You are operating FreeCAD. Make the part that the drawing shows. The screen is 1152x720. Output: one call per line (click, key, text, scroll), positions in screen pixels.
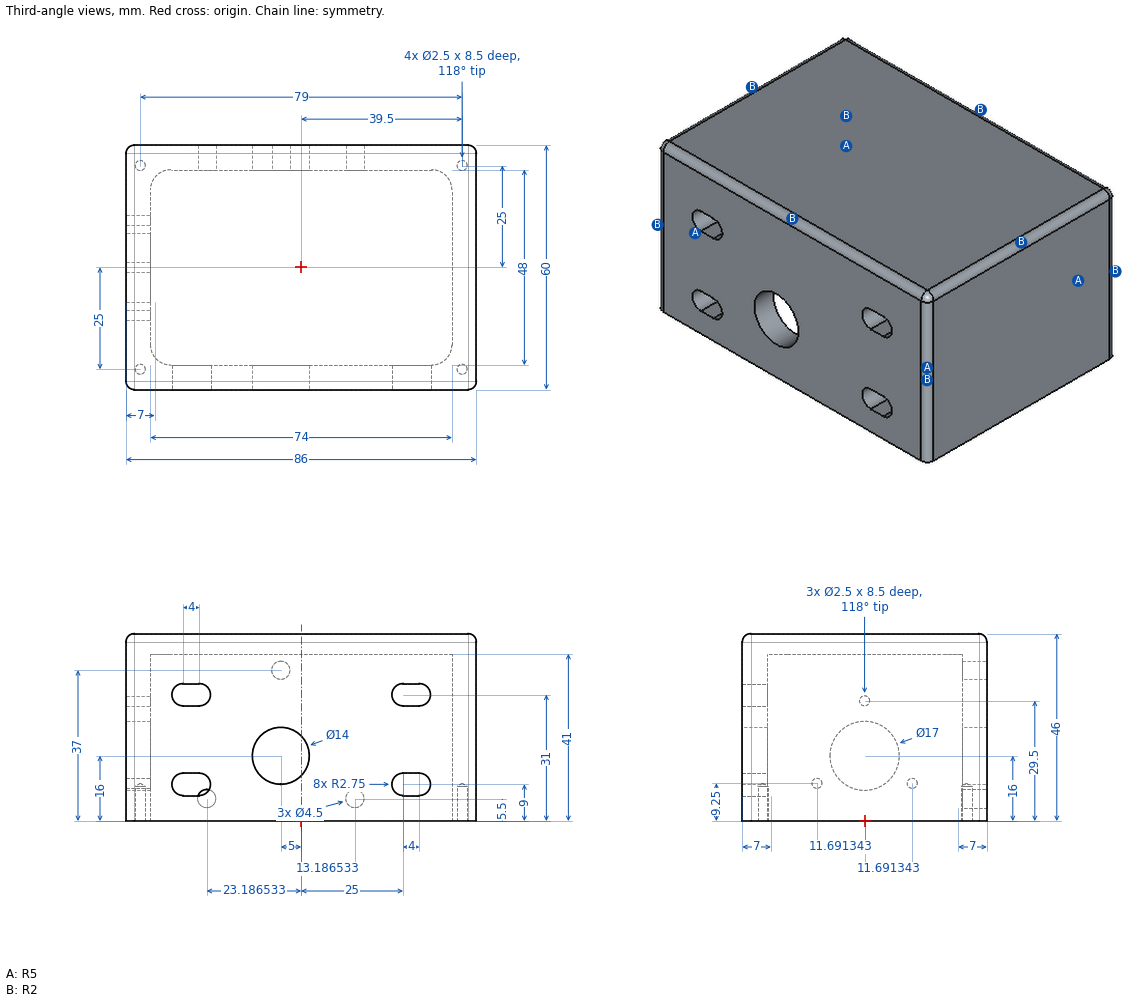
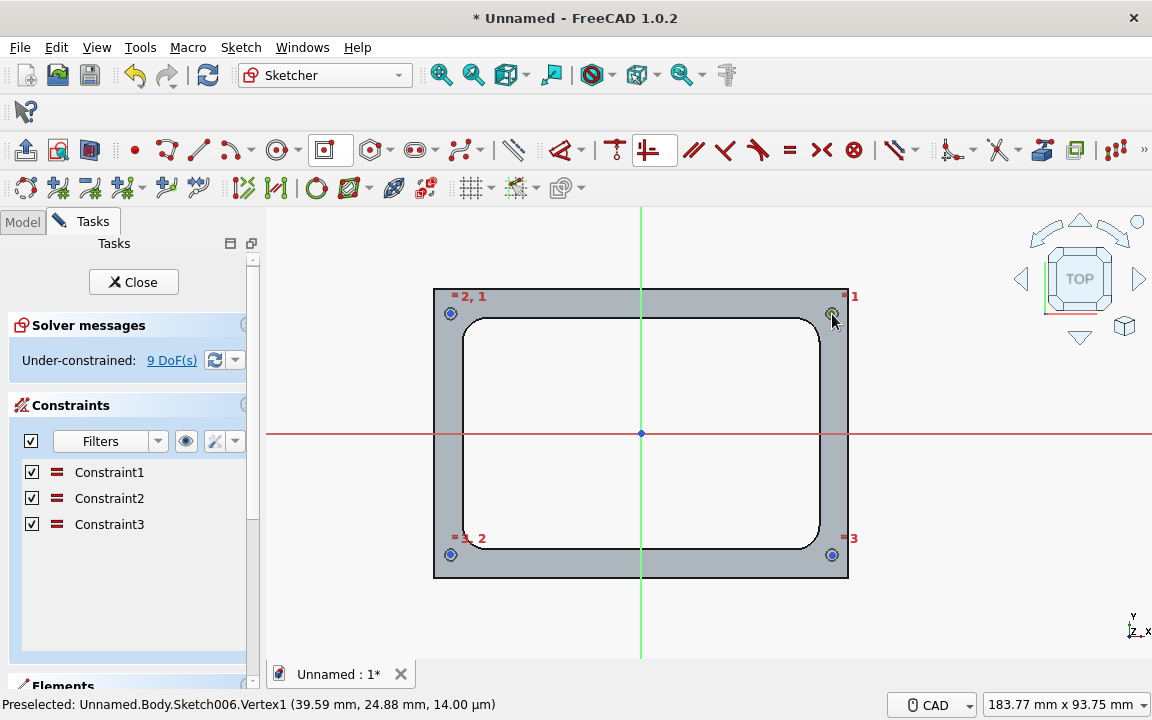
click(451, 314)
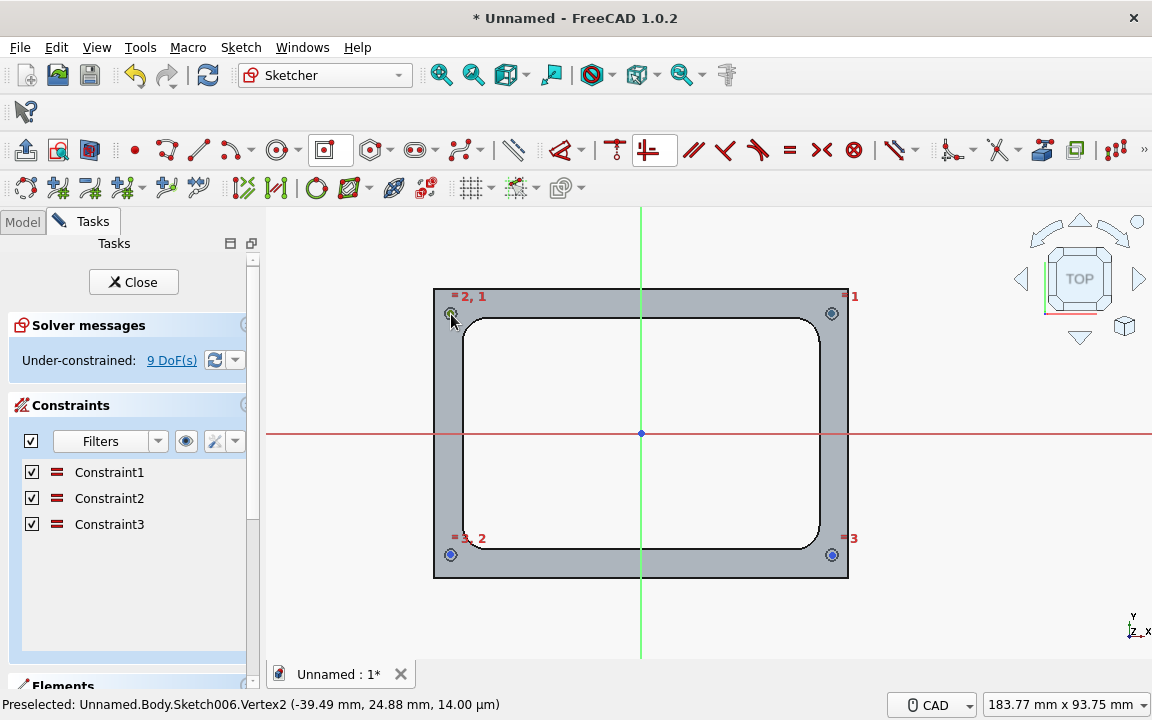
key(h)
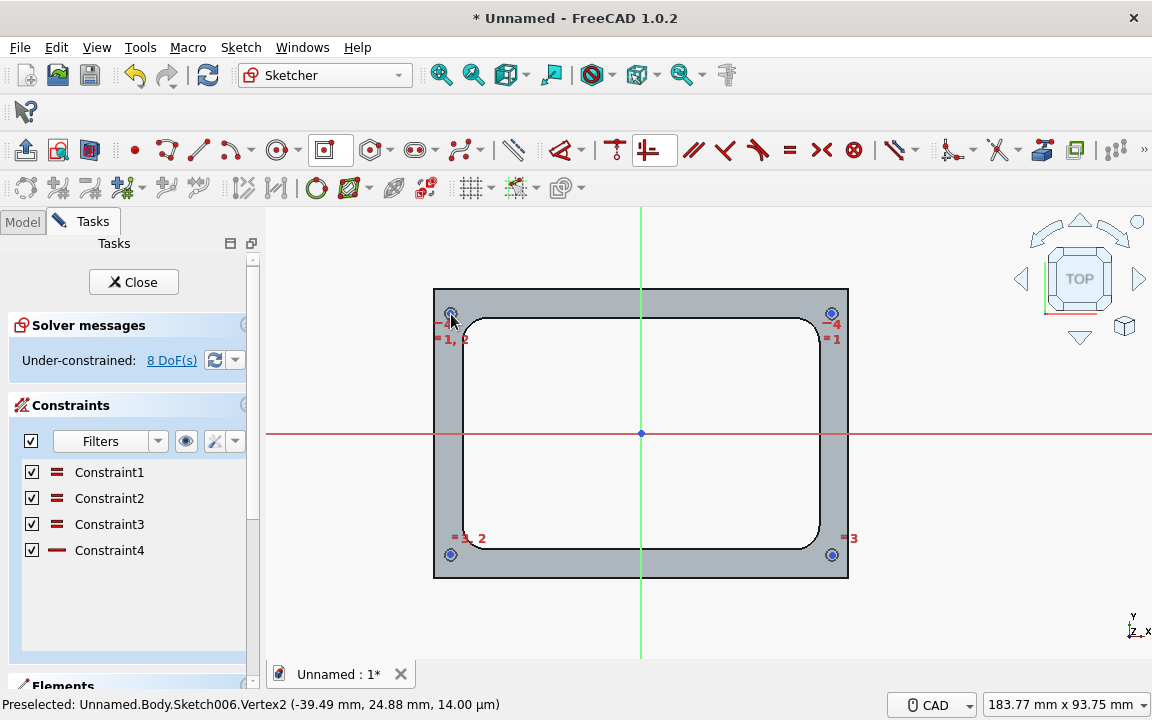
click(451, 314)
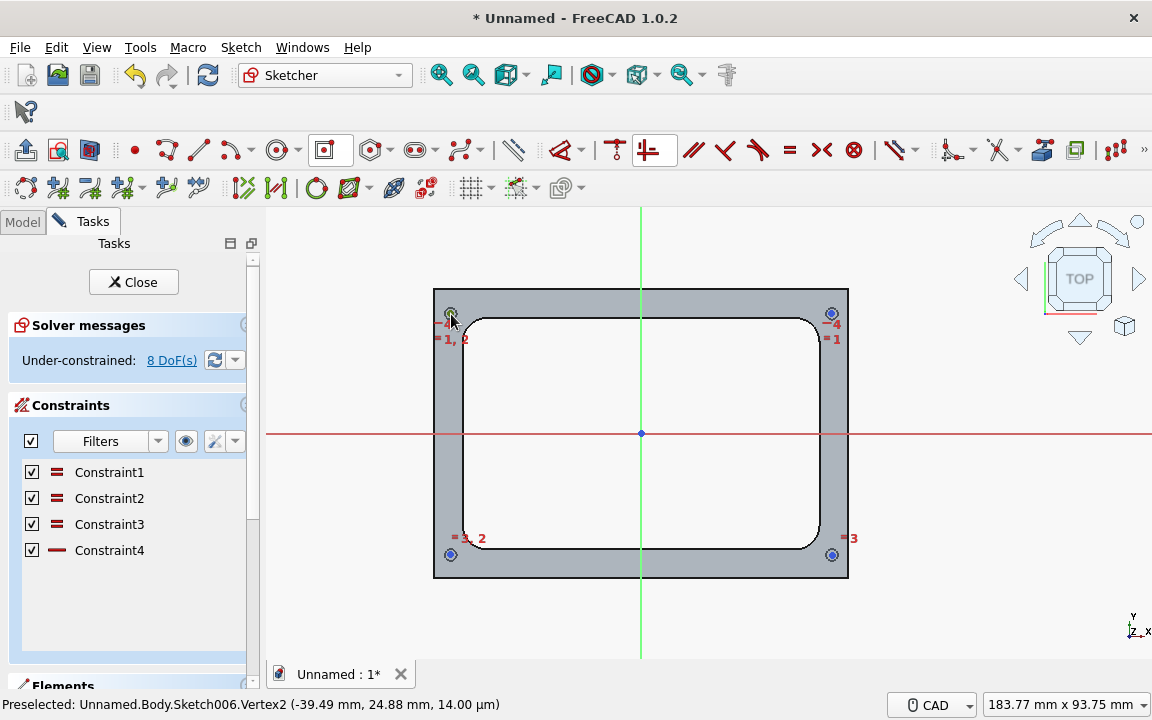
click(451, 555)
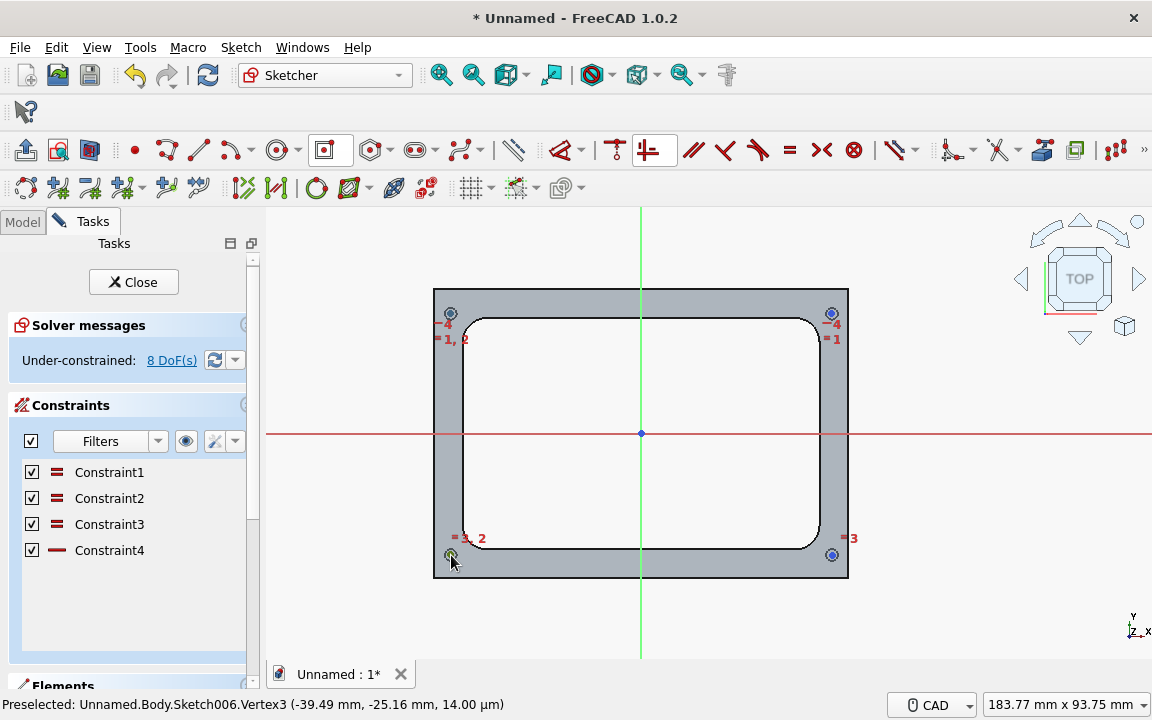
key(v)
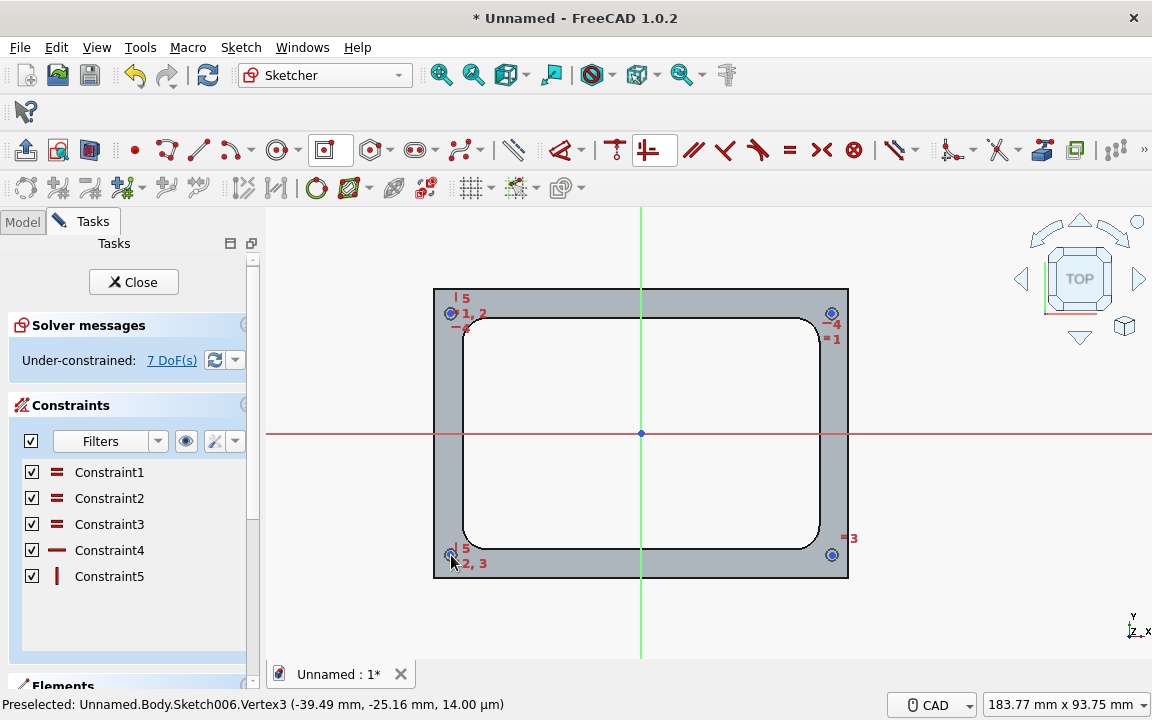
click(832, 314)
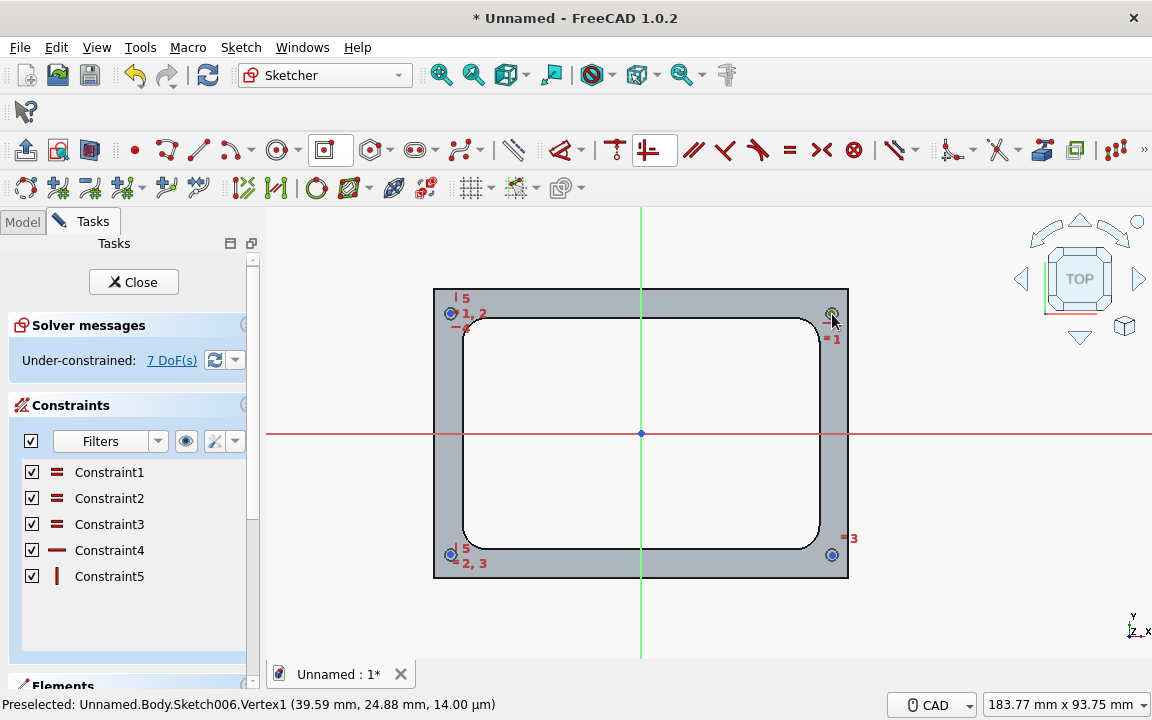
click(832, 555)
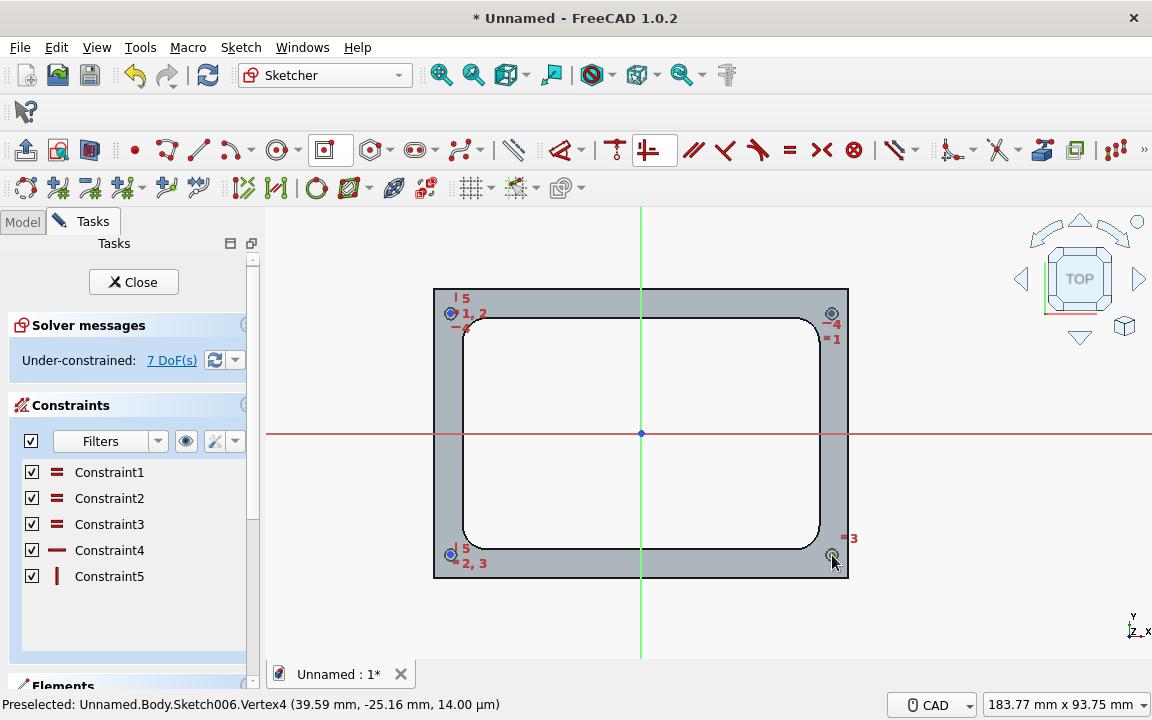
key(v)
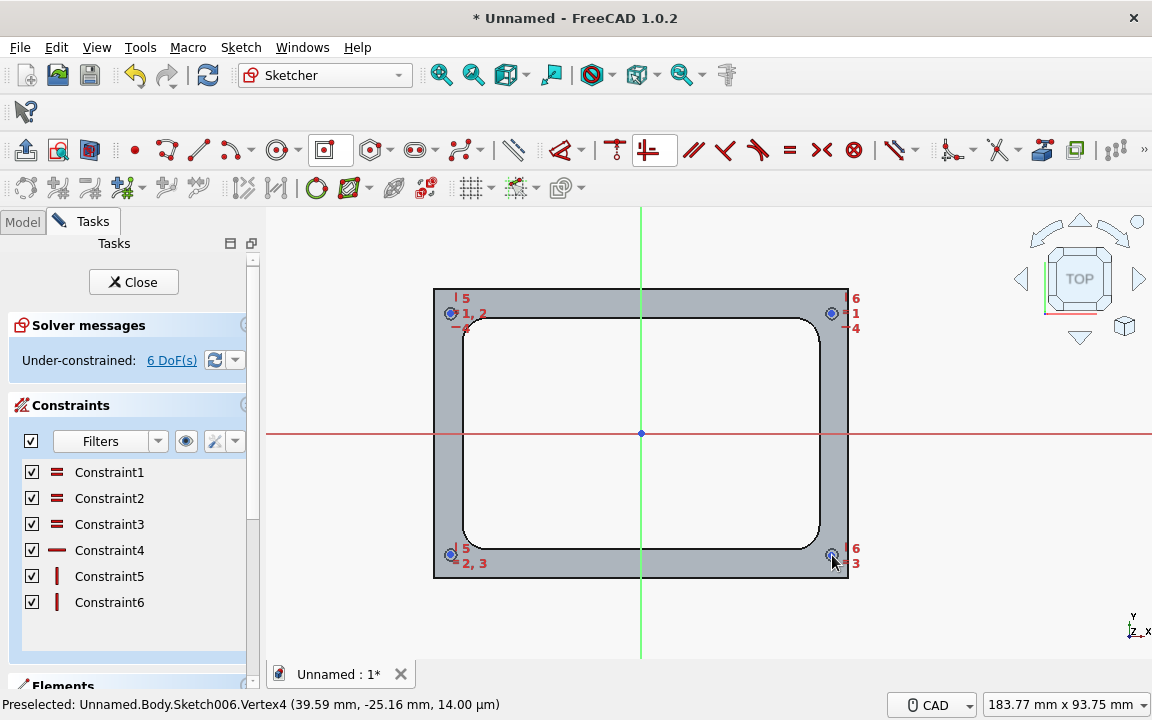
click(449, 557)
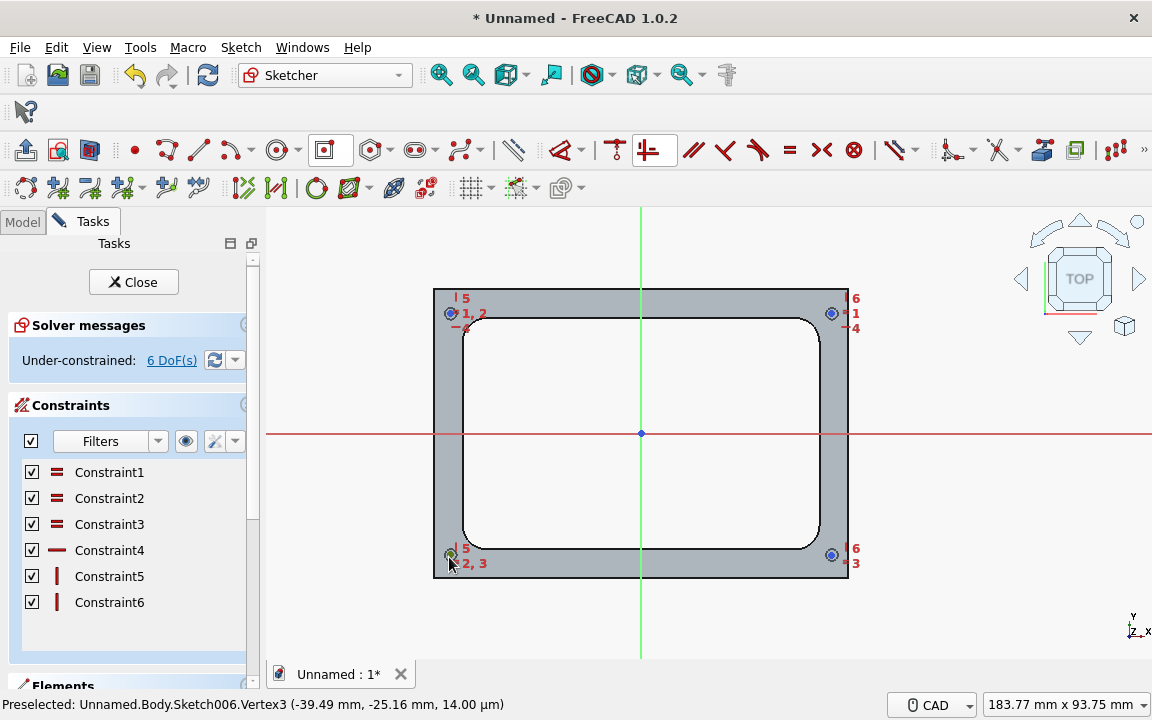
click(832, 555)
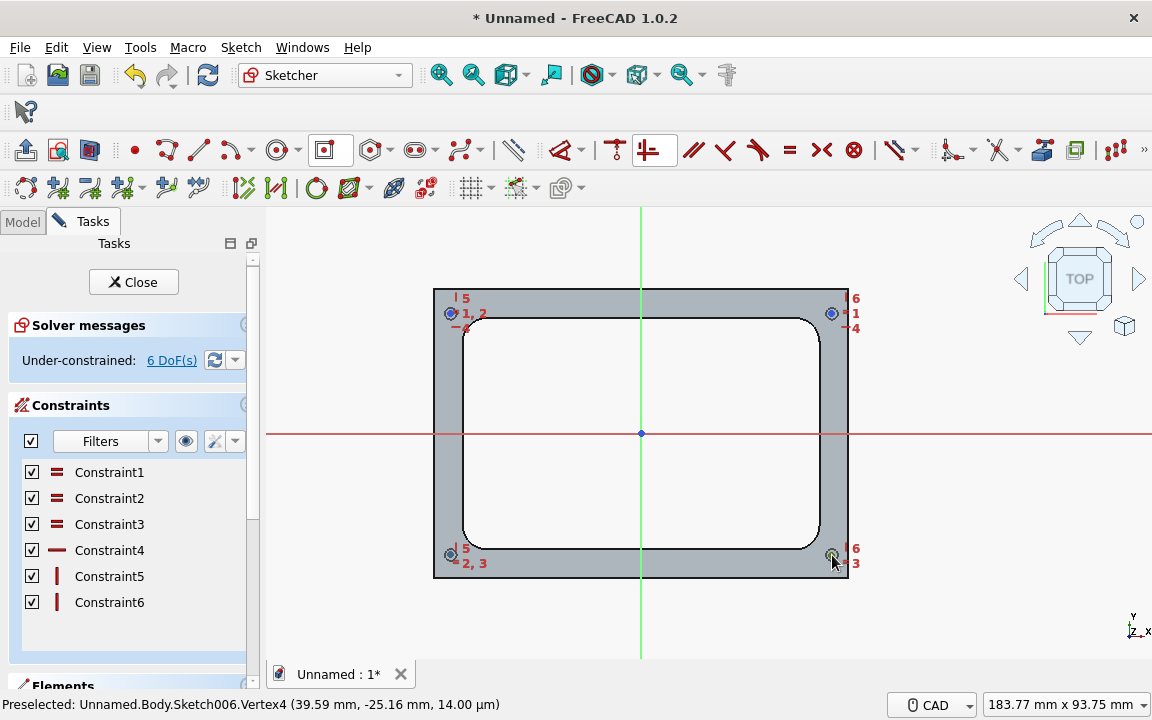
key(h)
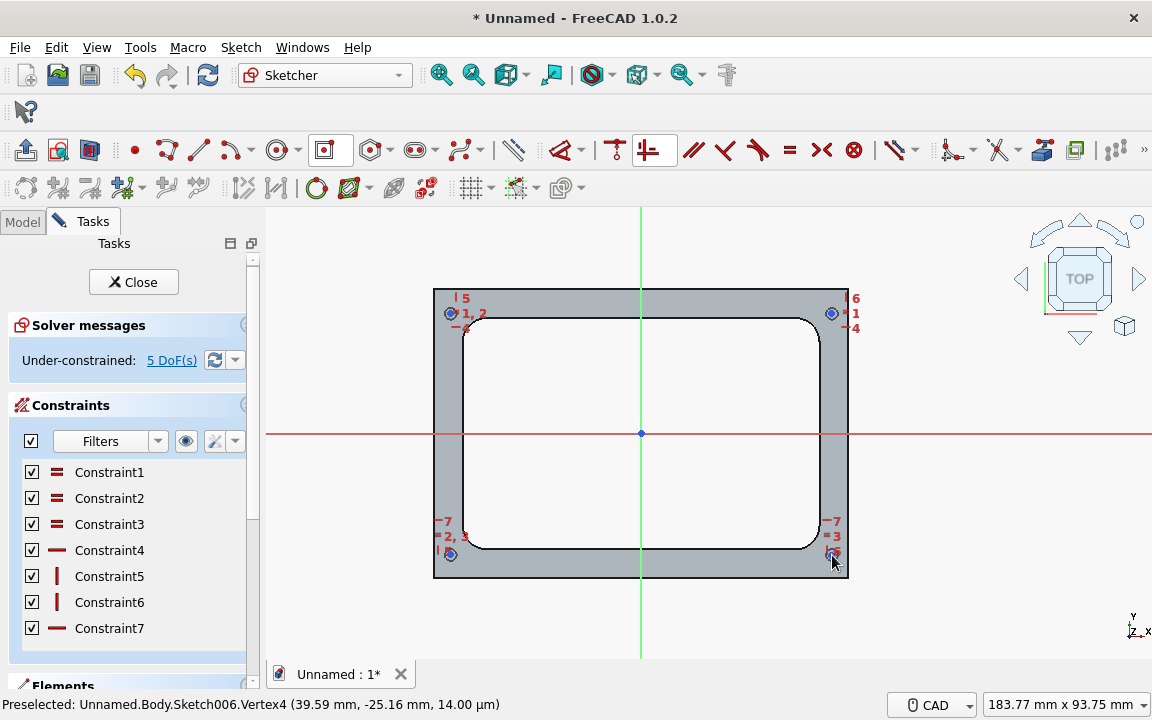
key(d)